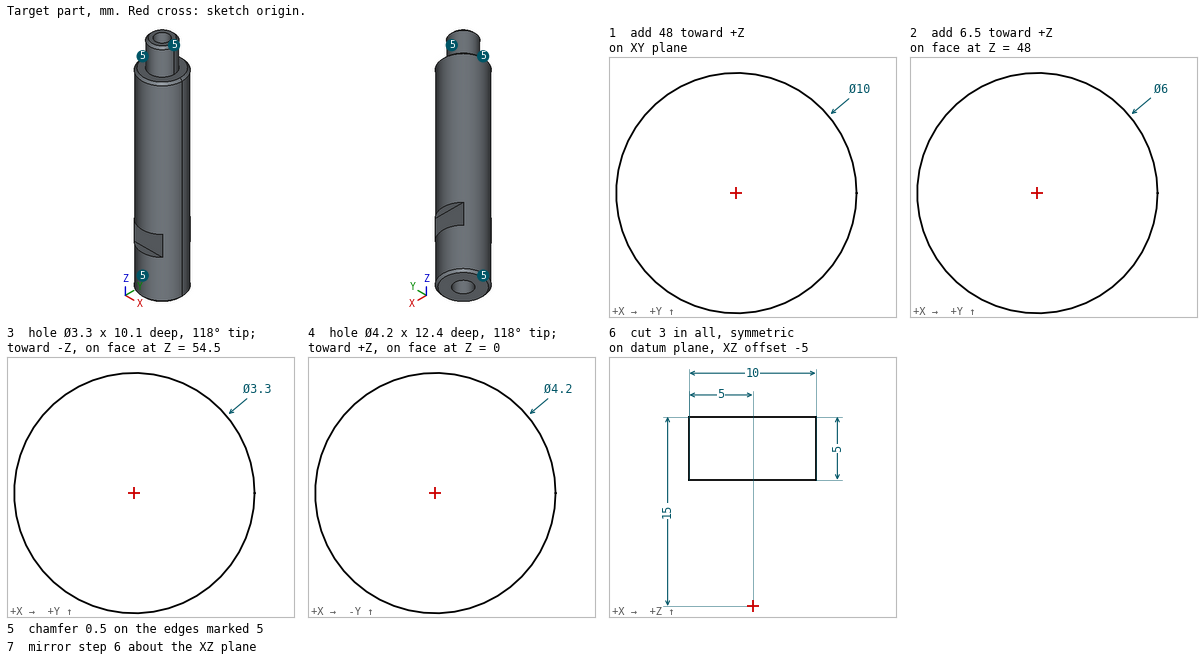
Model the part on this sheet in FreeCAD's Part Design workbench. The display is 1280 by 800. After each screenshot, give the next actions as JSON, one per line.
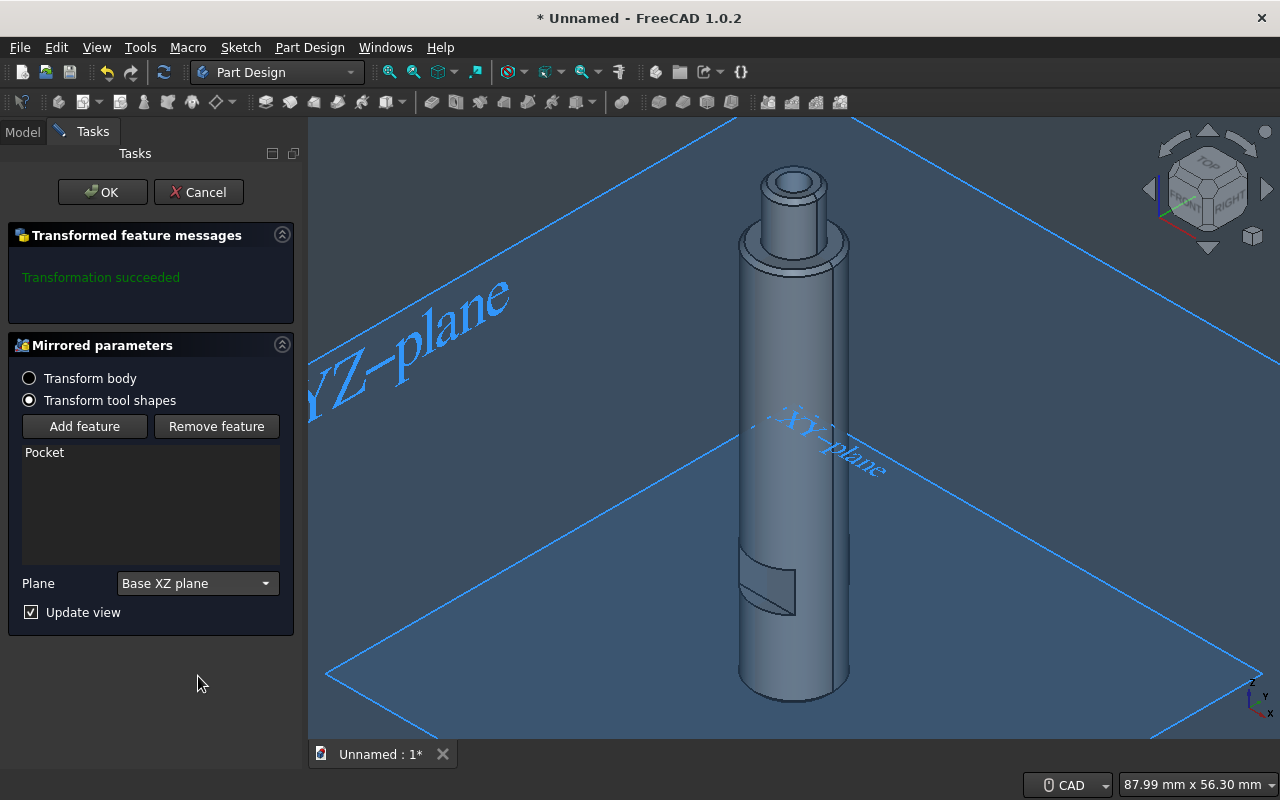
{"action": "left_click", "coordinate": [103, 192]}